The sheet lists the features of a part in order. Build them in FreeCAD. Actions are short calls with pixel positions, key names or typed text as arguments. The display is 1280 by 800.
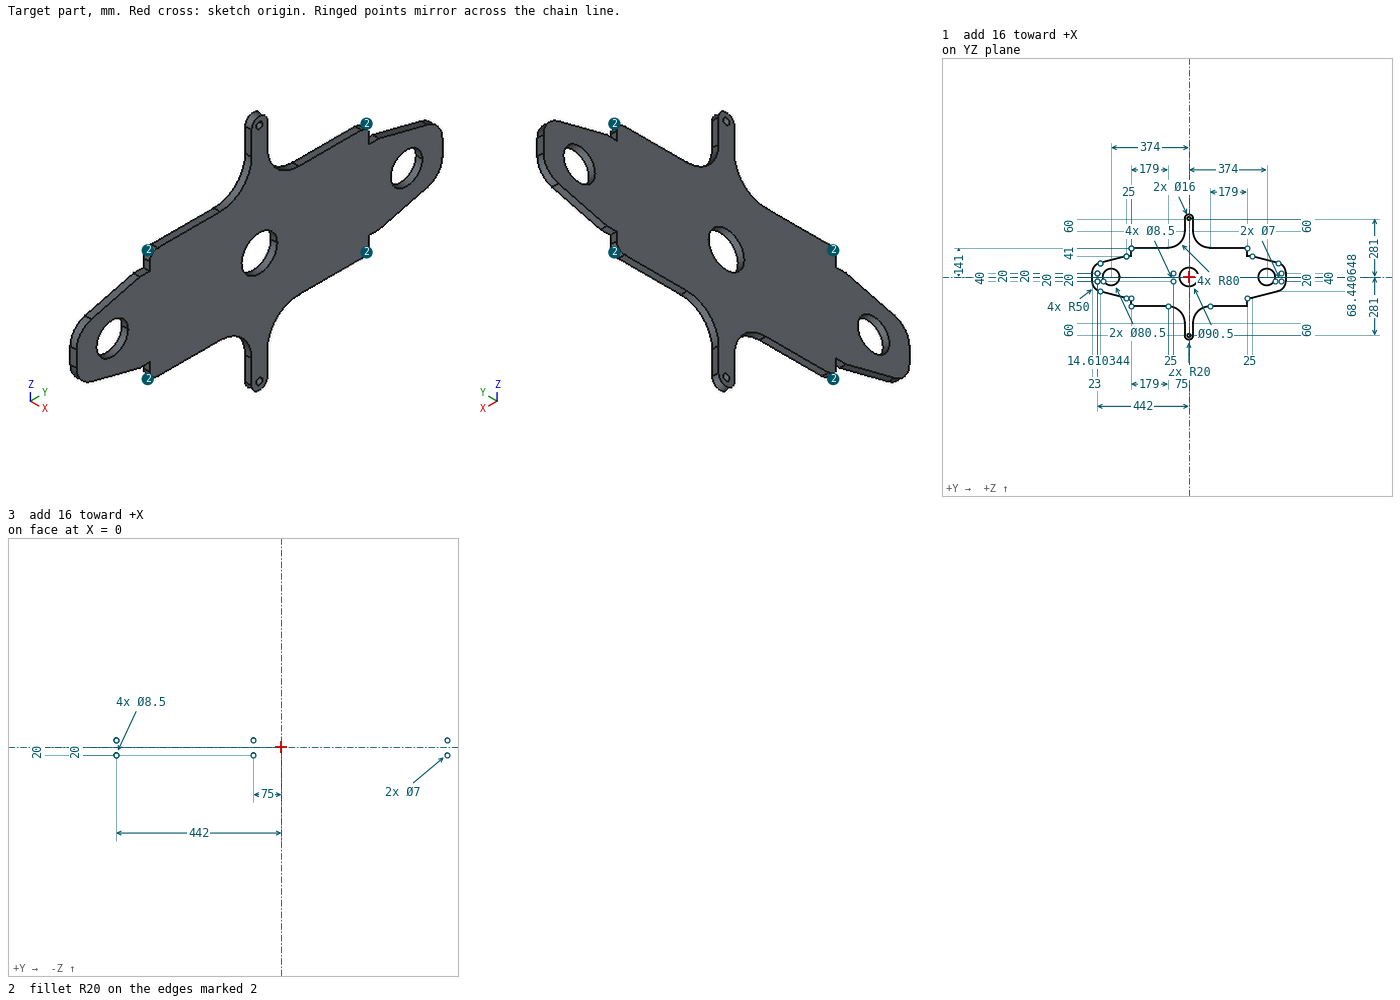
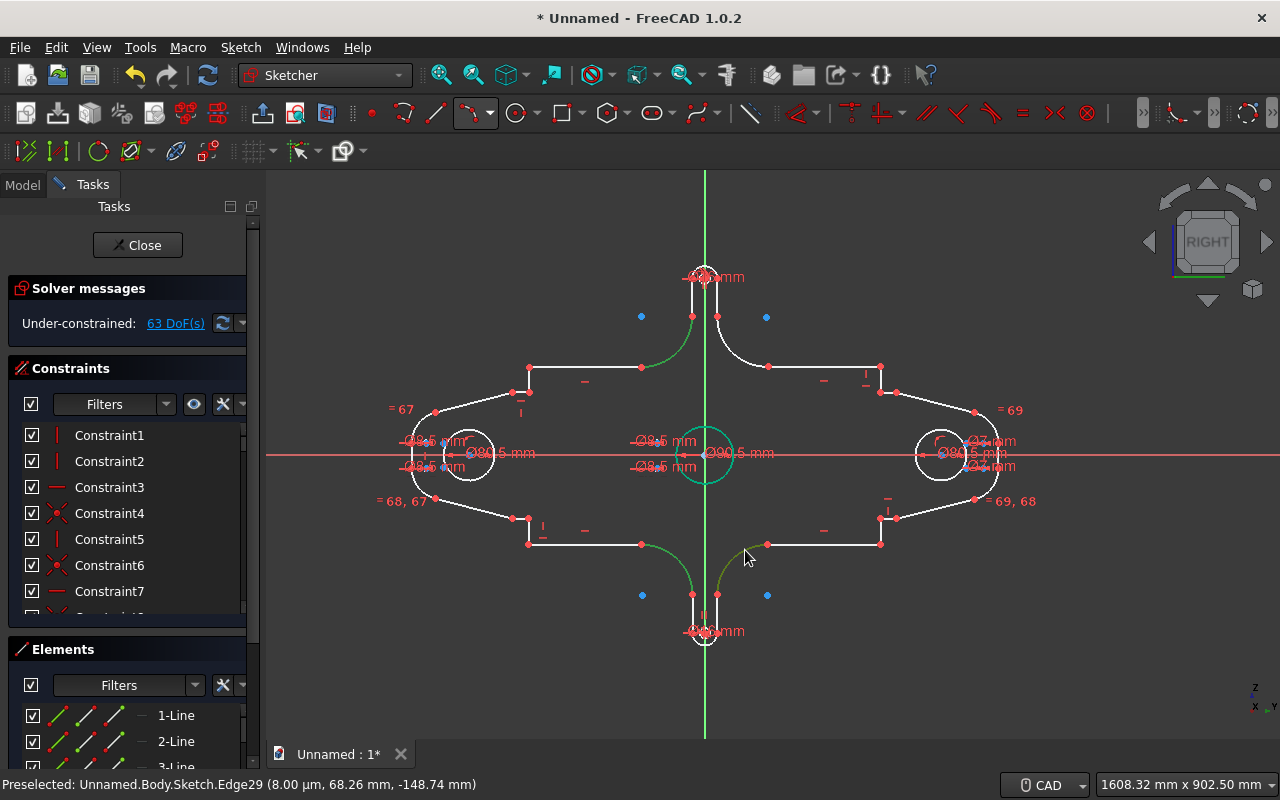
click(723, 339)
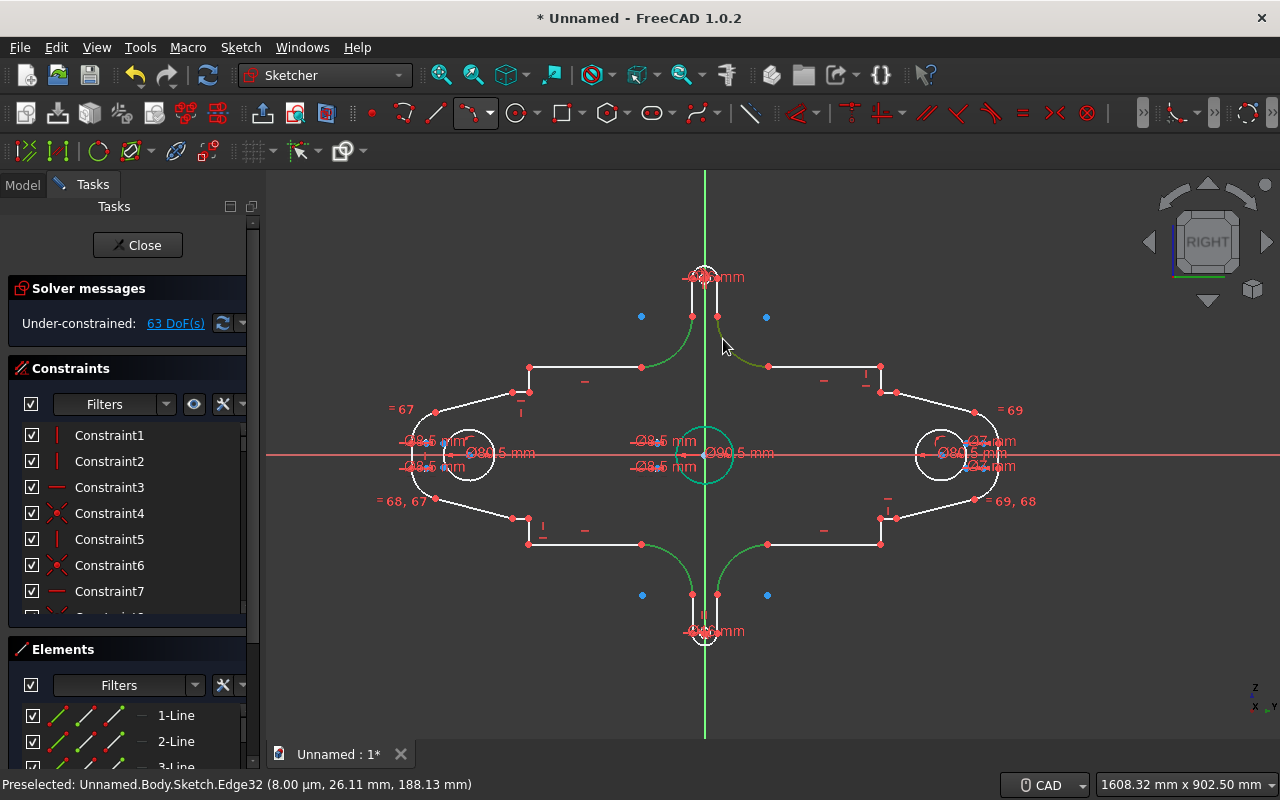
click(1024, 114)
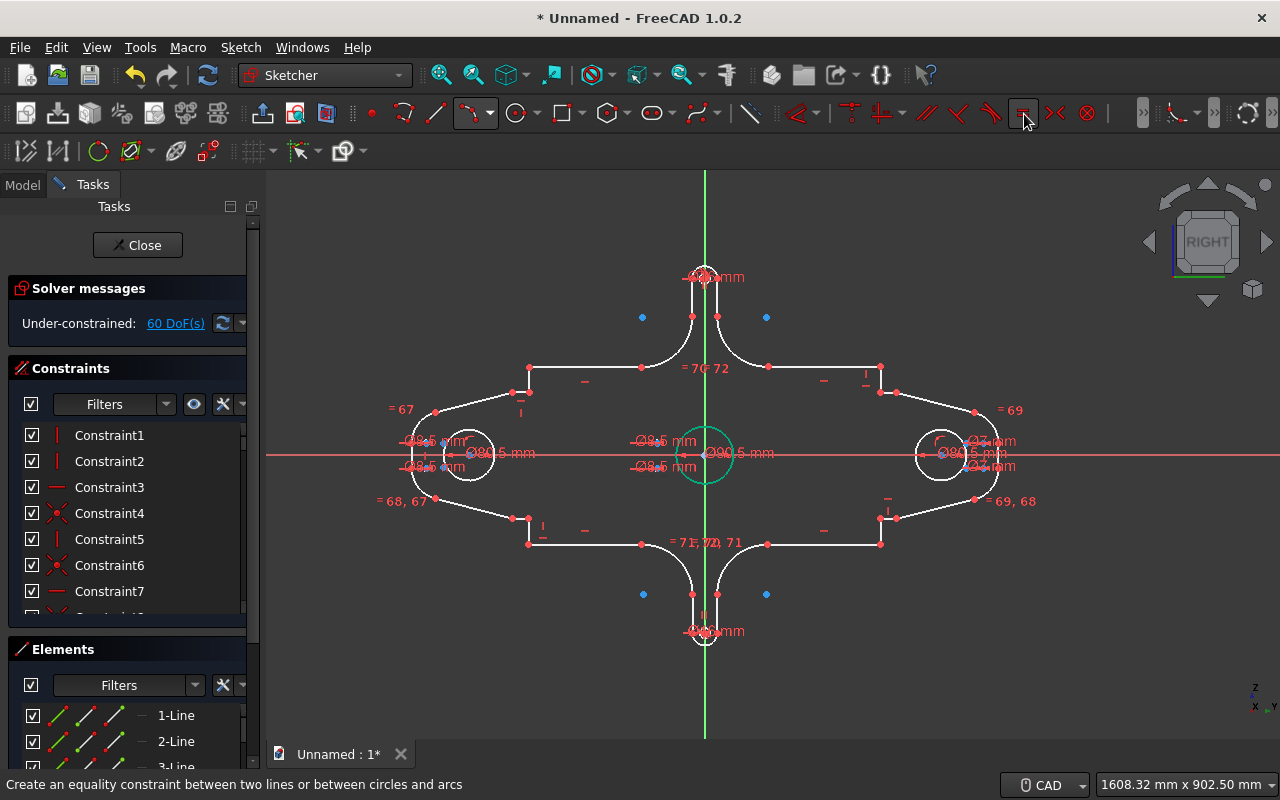
scroll(705, 266, up, 3)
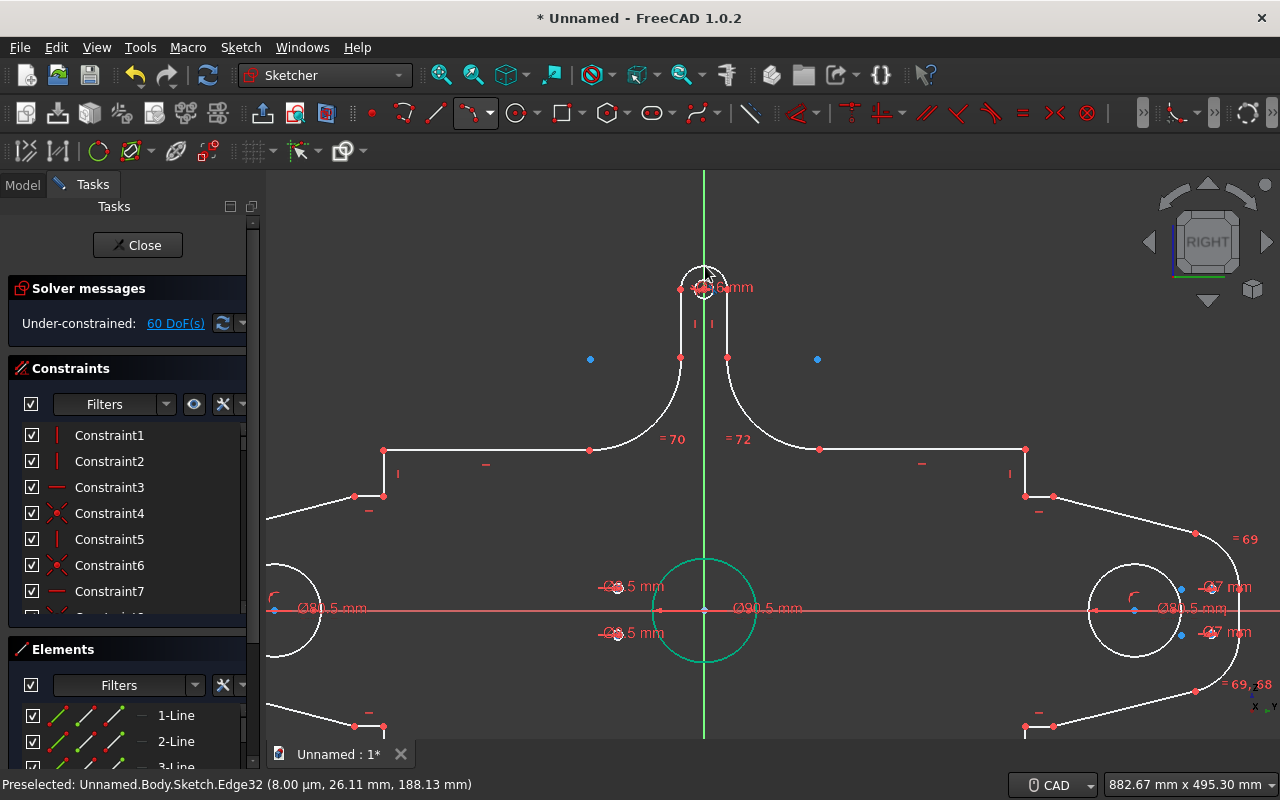
click(704, 266)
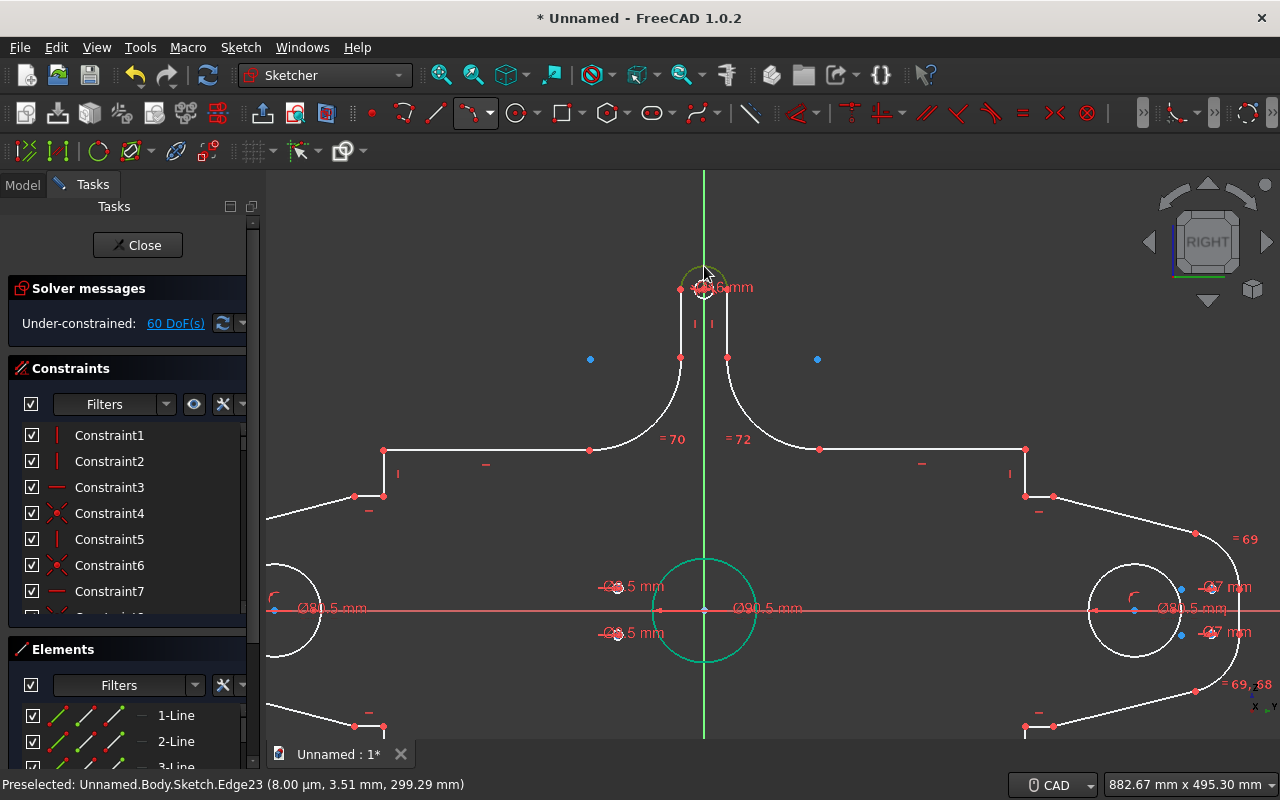
scroll(705, 265, down, 3)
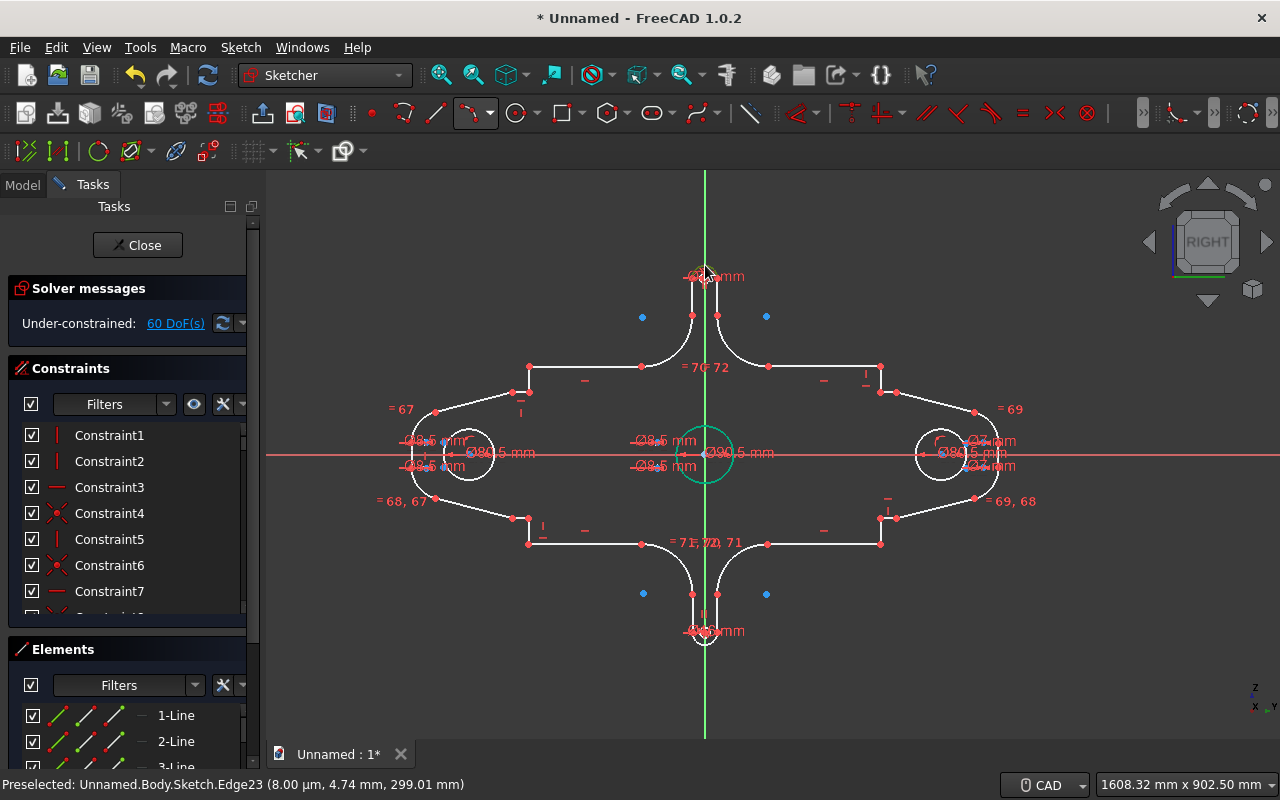
scroll(698, 643, up, 4)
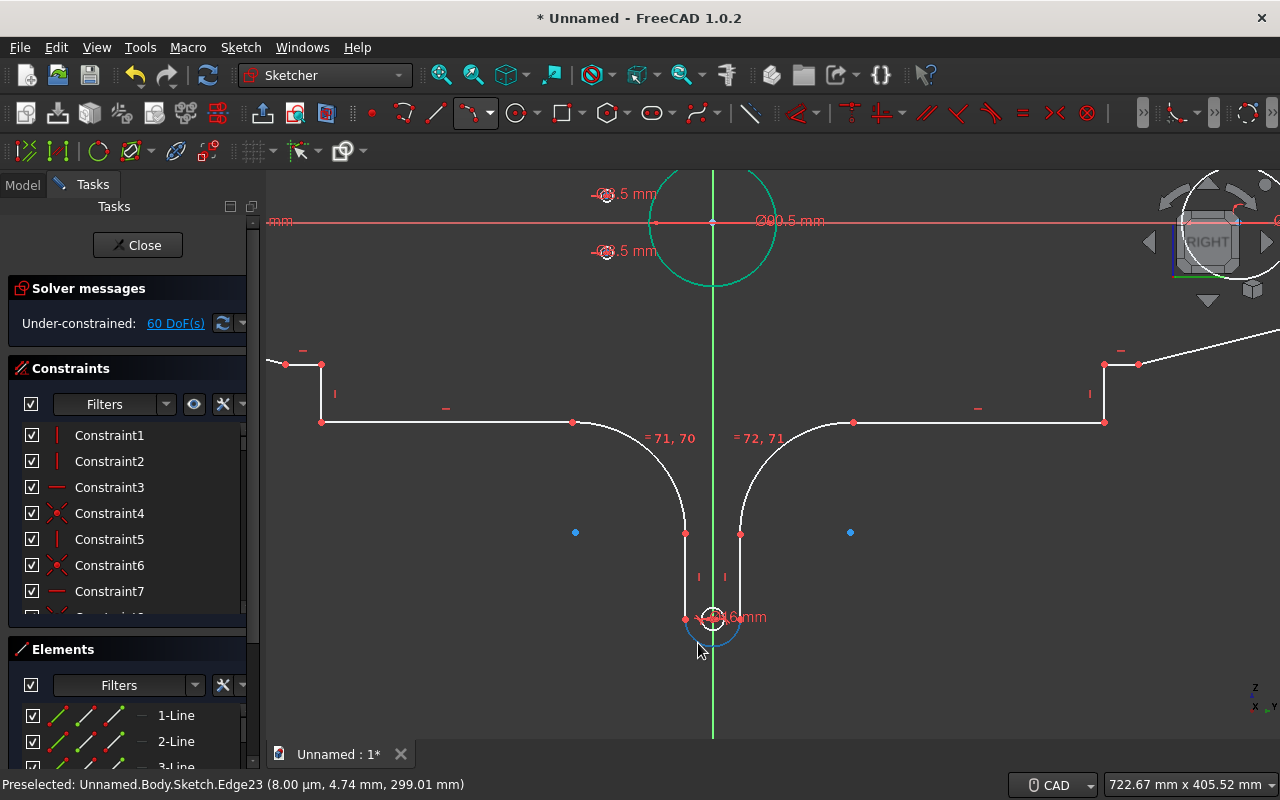
click(697, 641)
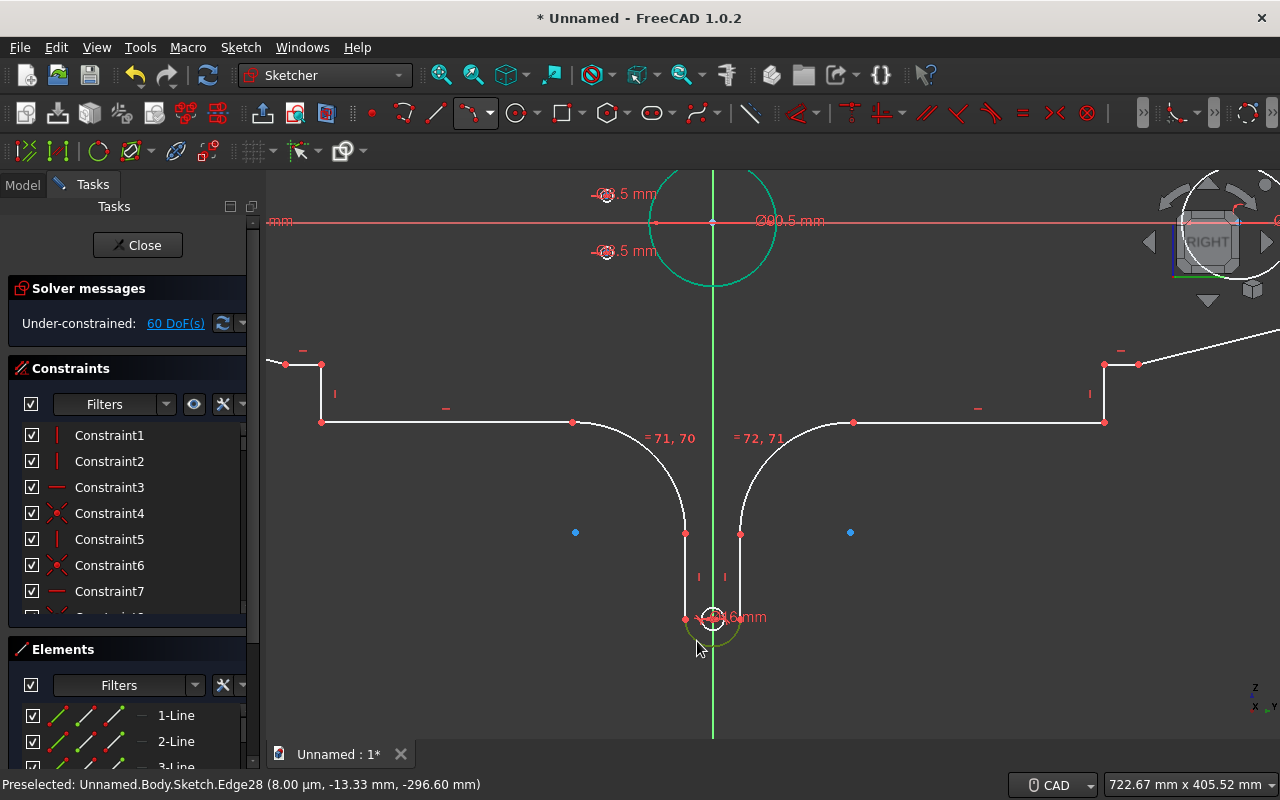
click(1024, 114)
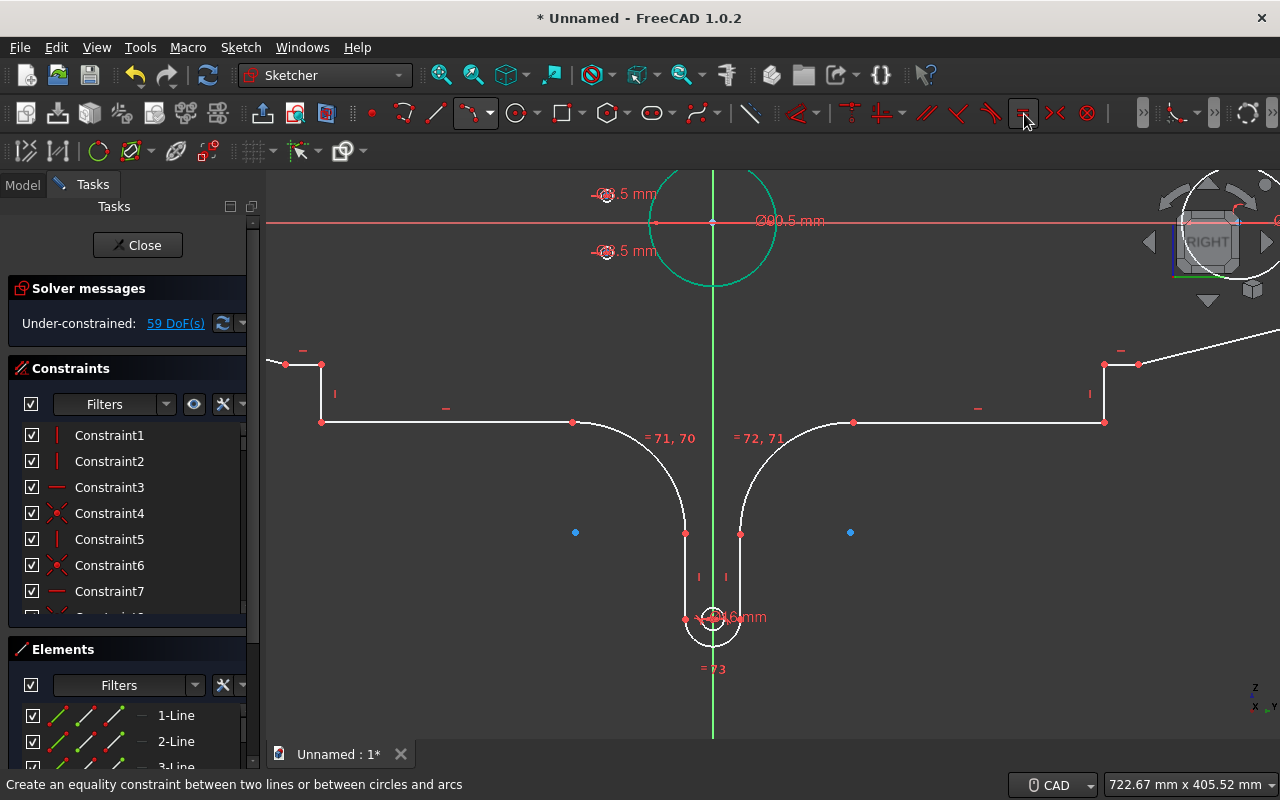
scroll(698, 643, down, 4)